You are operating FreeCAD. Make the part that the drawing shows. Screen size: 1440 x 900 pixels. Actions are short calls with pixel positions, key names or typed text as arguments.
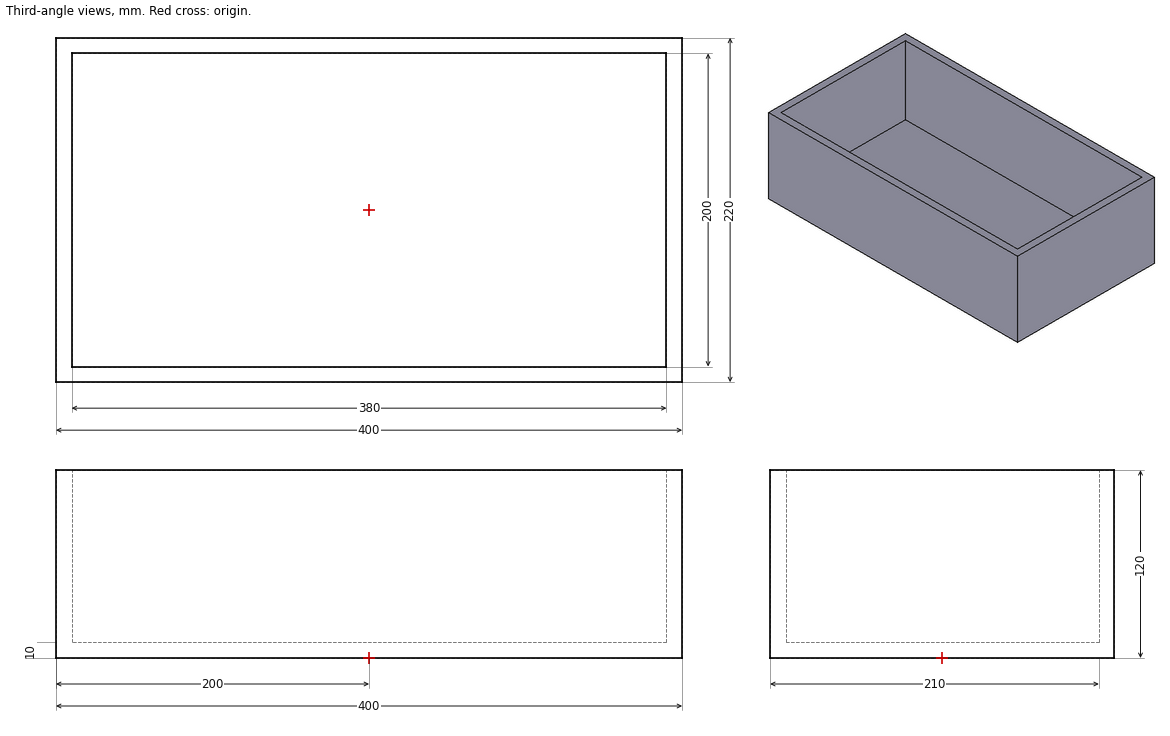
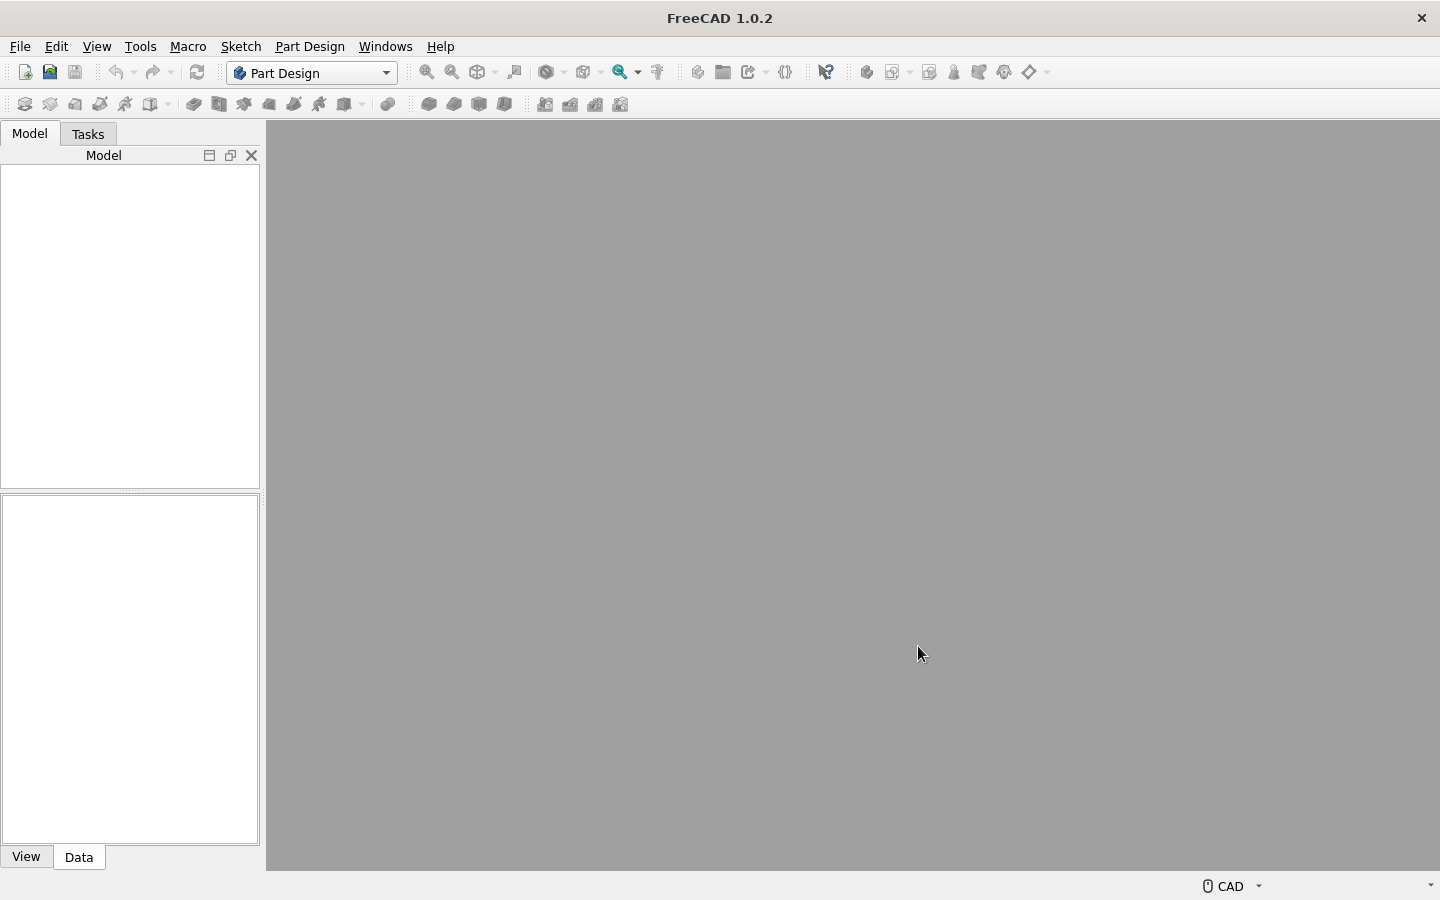
click(25, 72)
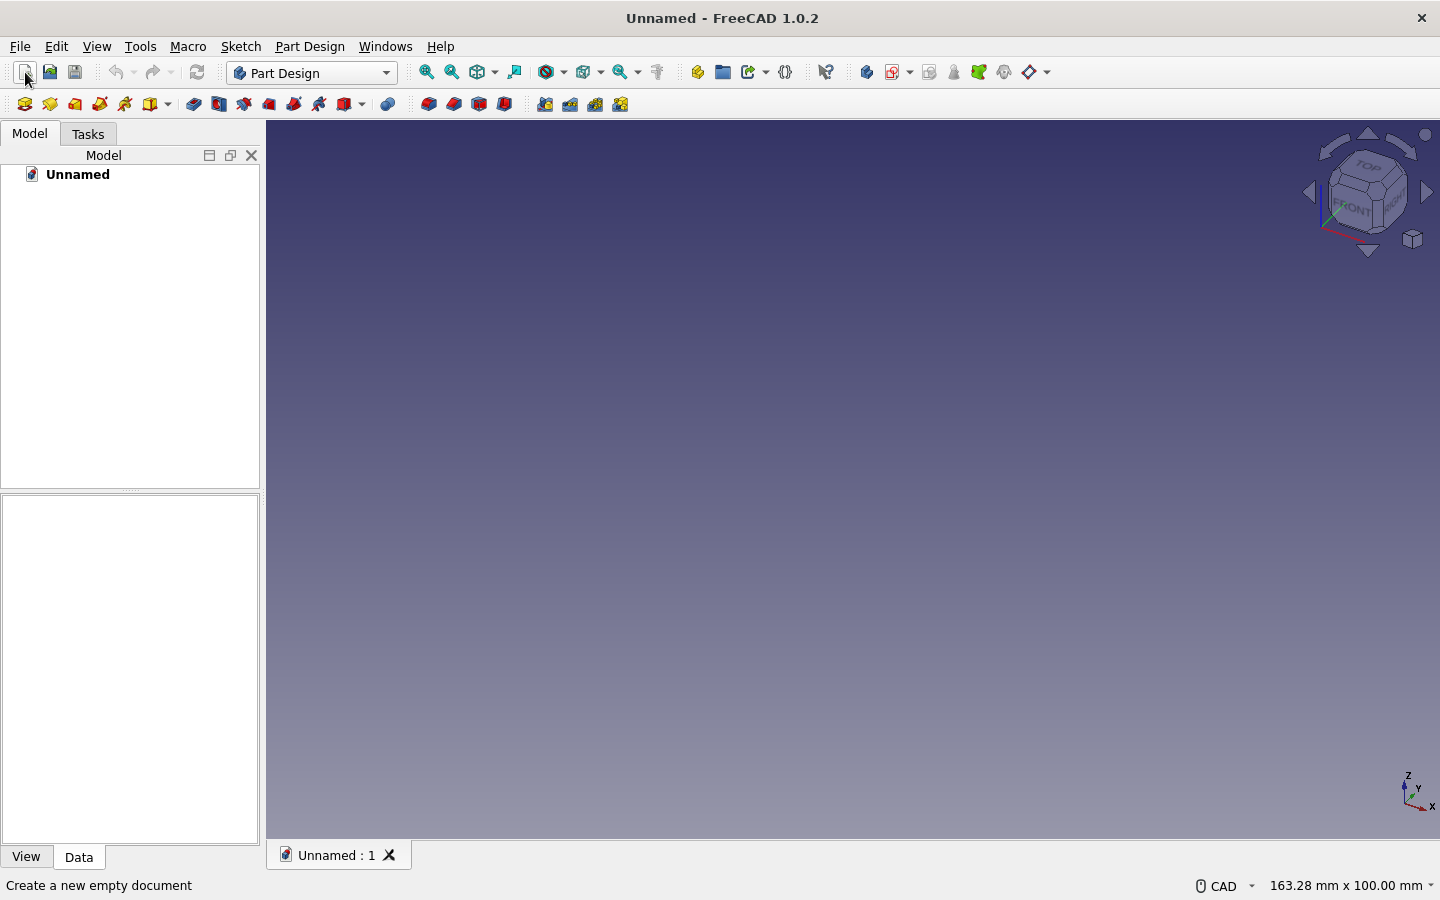
click(892, 72)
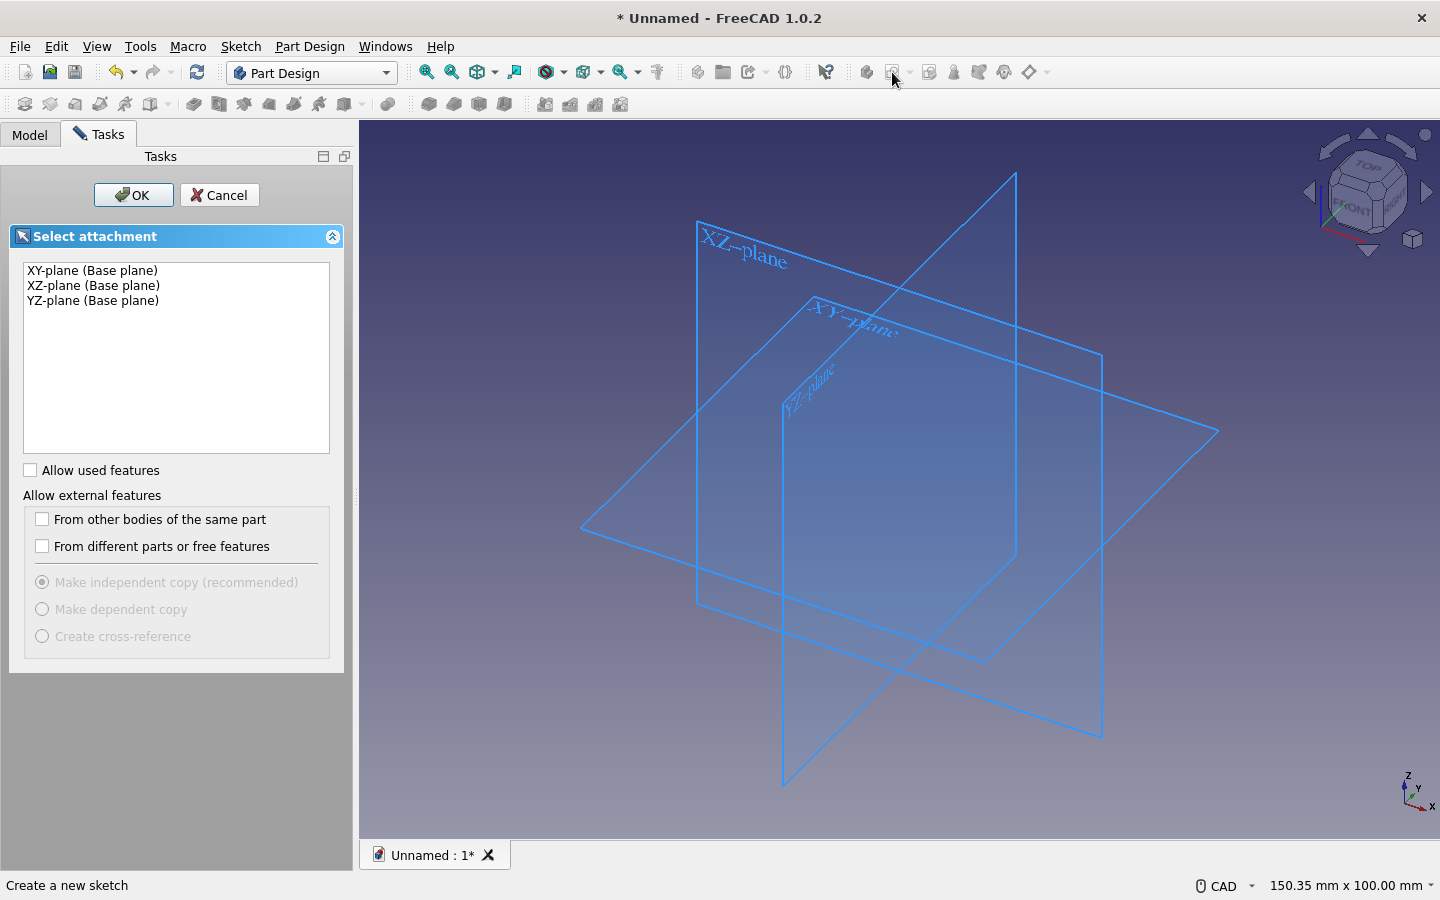
click(84, 270)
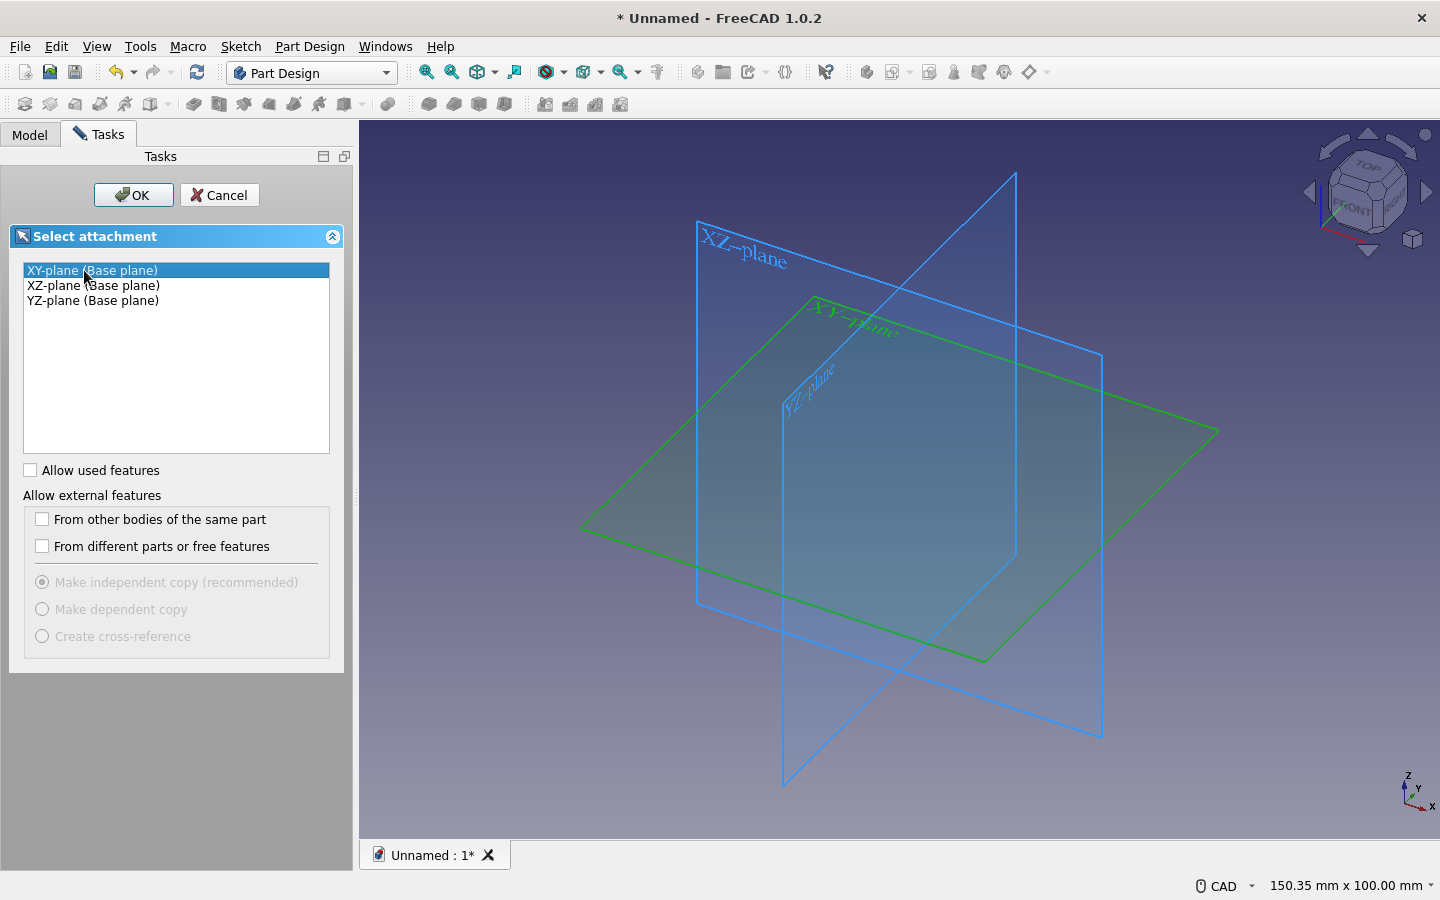
click(134, 195)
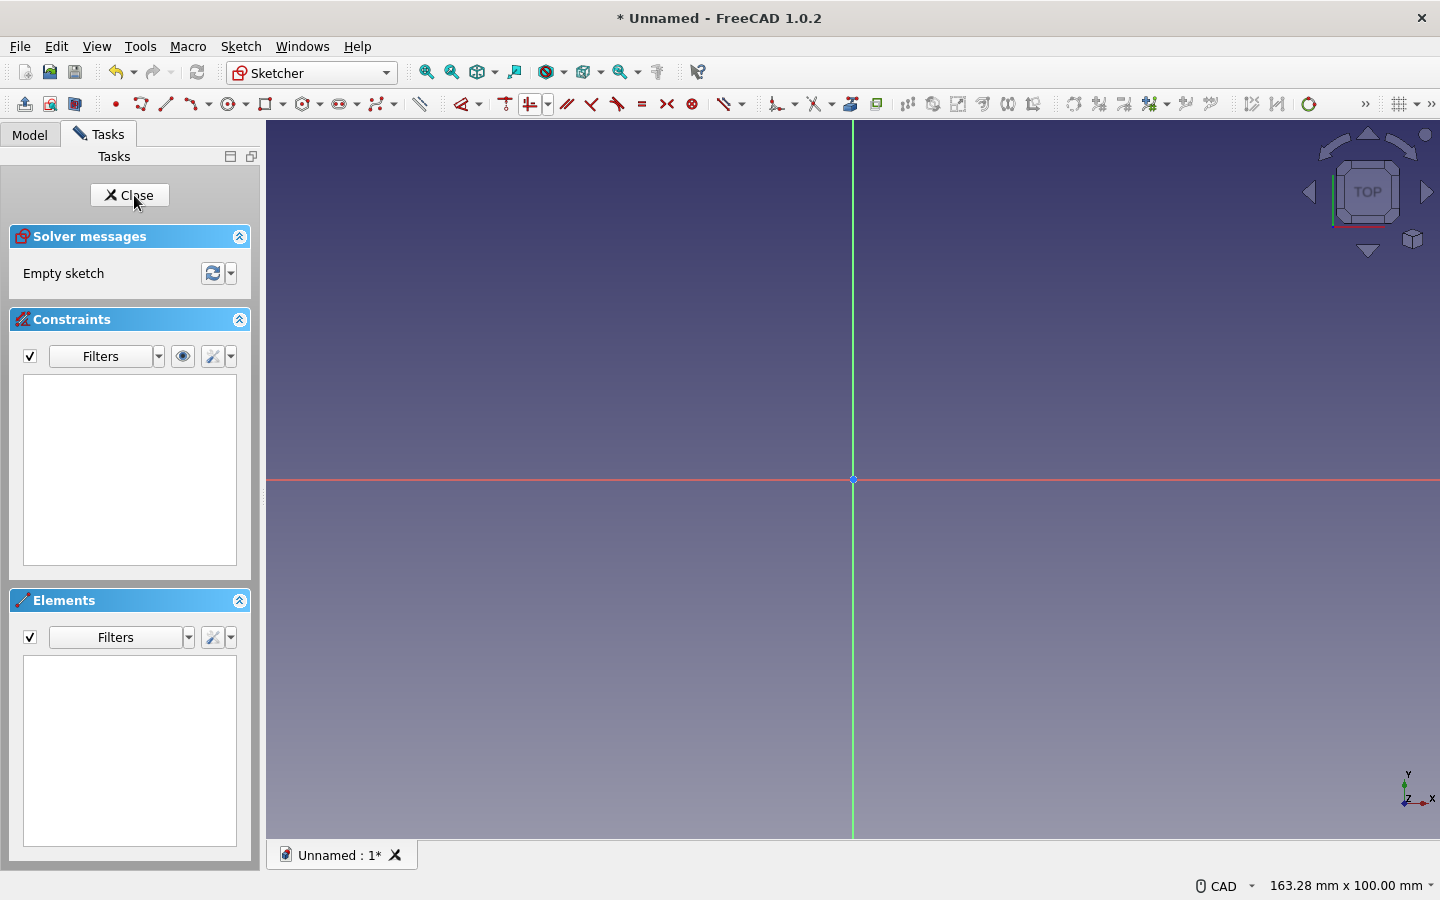
scroll(762, 480, down, 7)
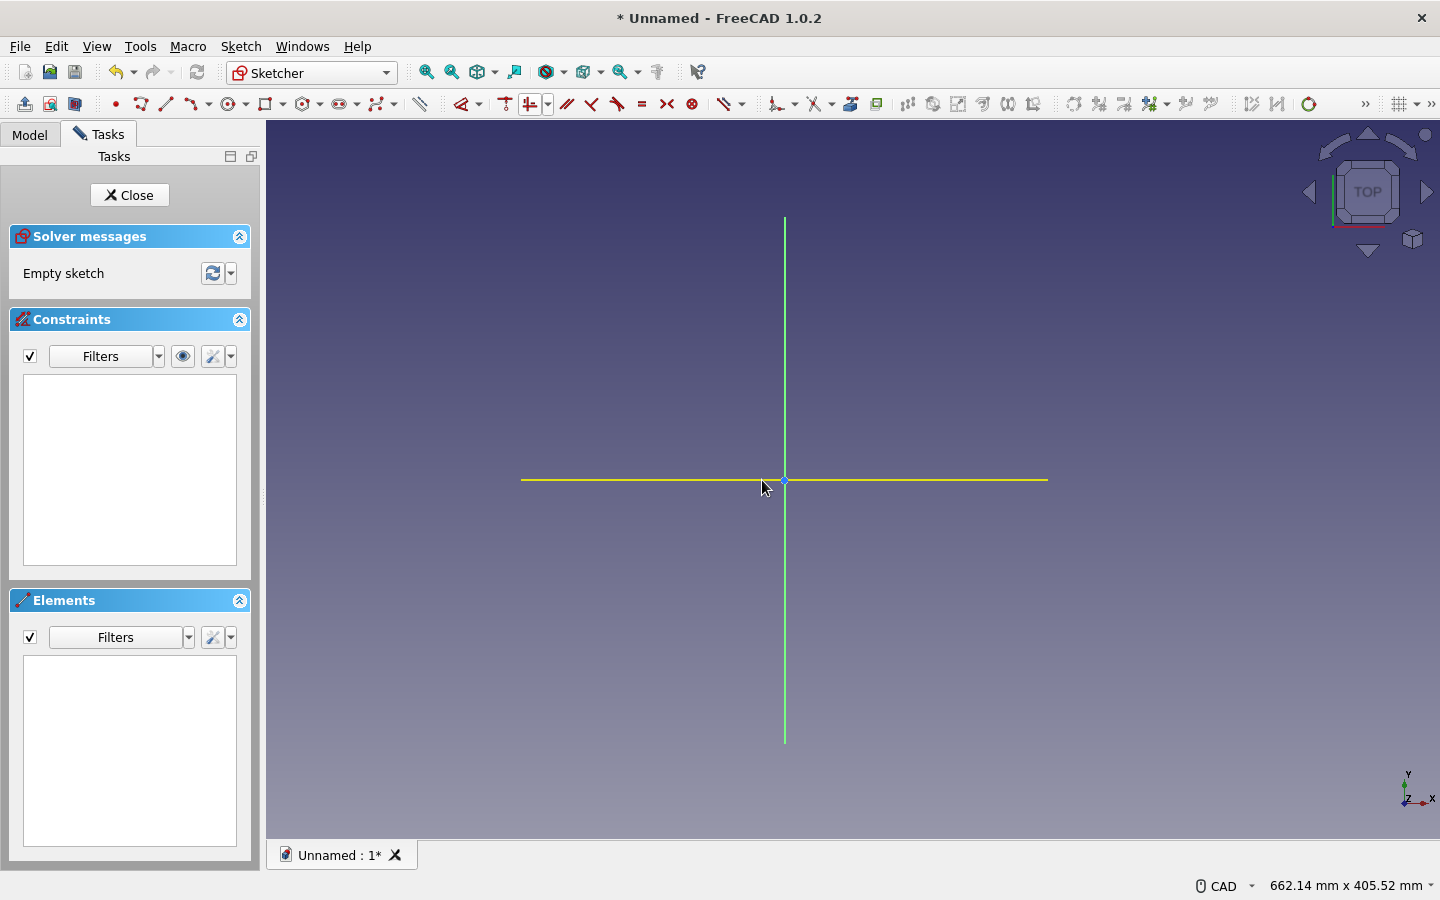
click(282, 104)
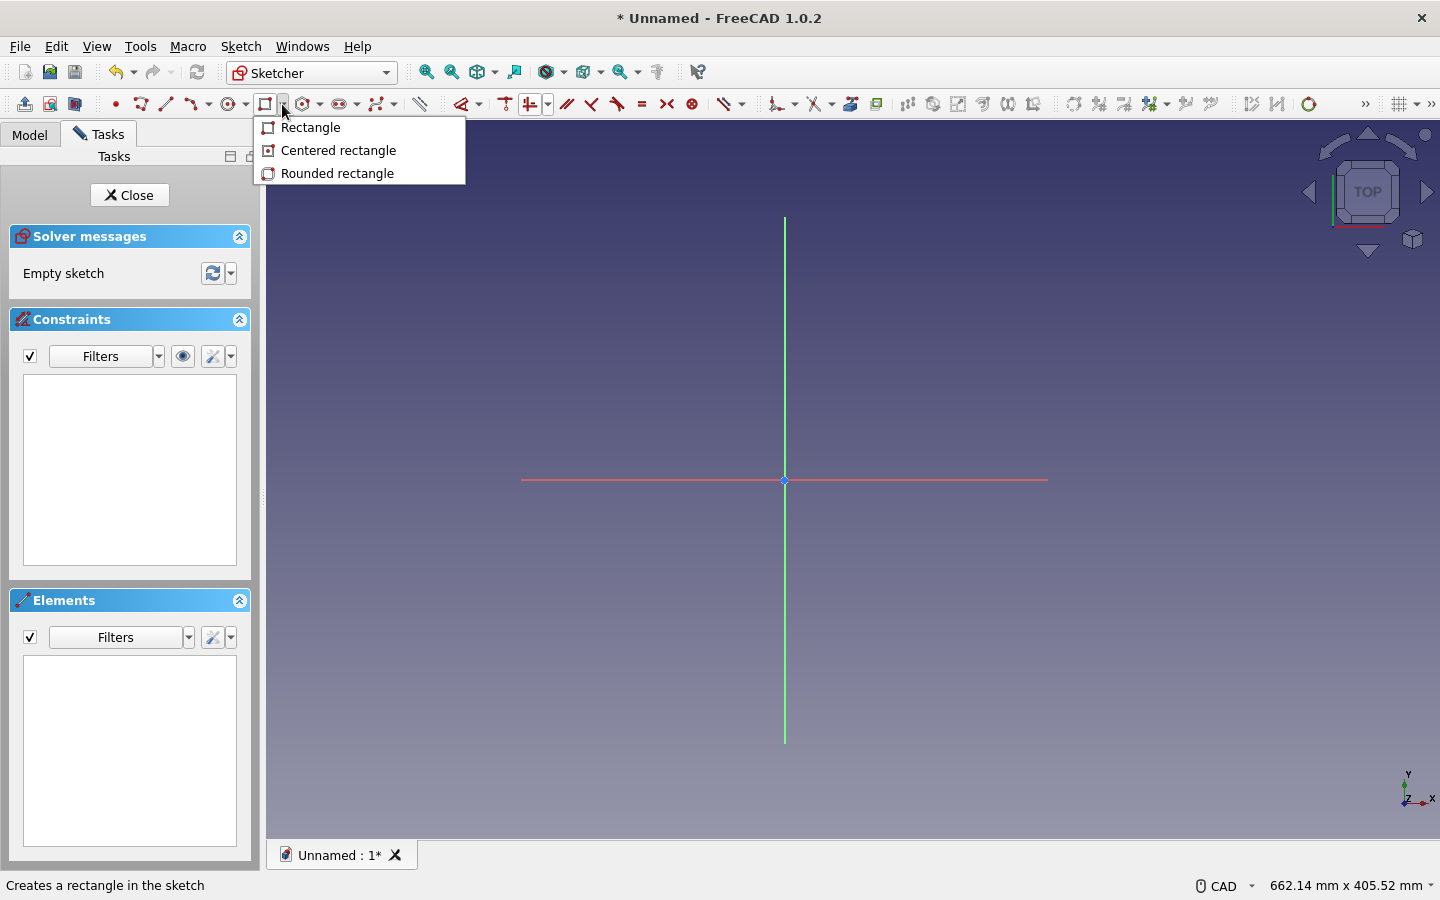
click(360, 150)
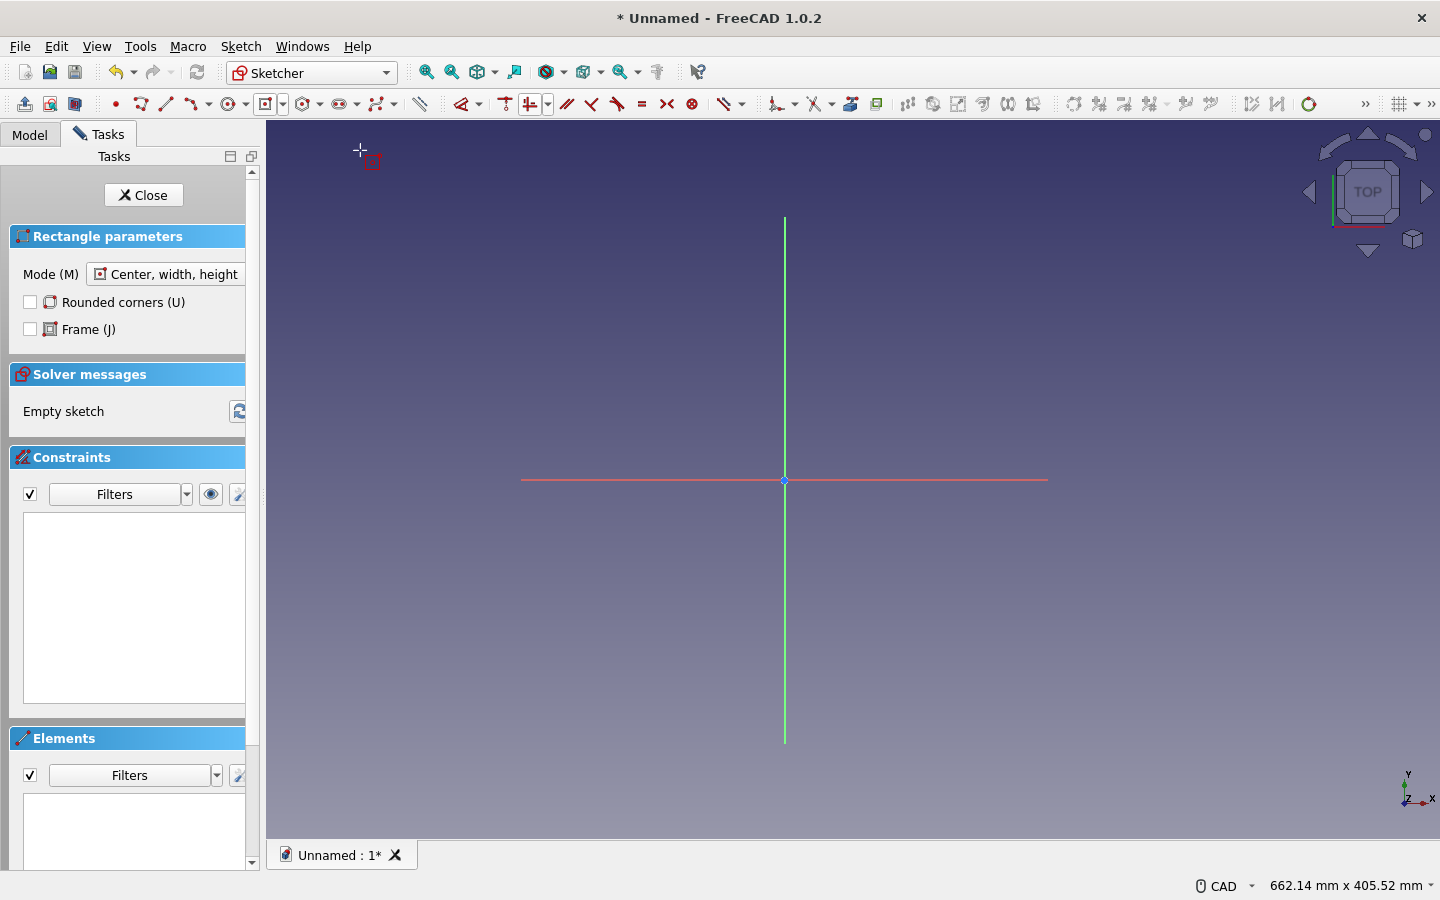
click(785, 480)
move(1139, 285)